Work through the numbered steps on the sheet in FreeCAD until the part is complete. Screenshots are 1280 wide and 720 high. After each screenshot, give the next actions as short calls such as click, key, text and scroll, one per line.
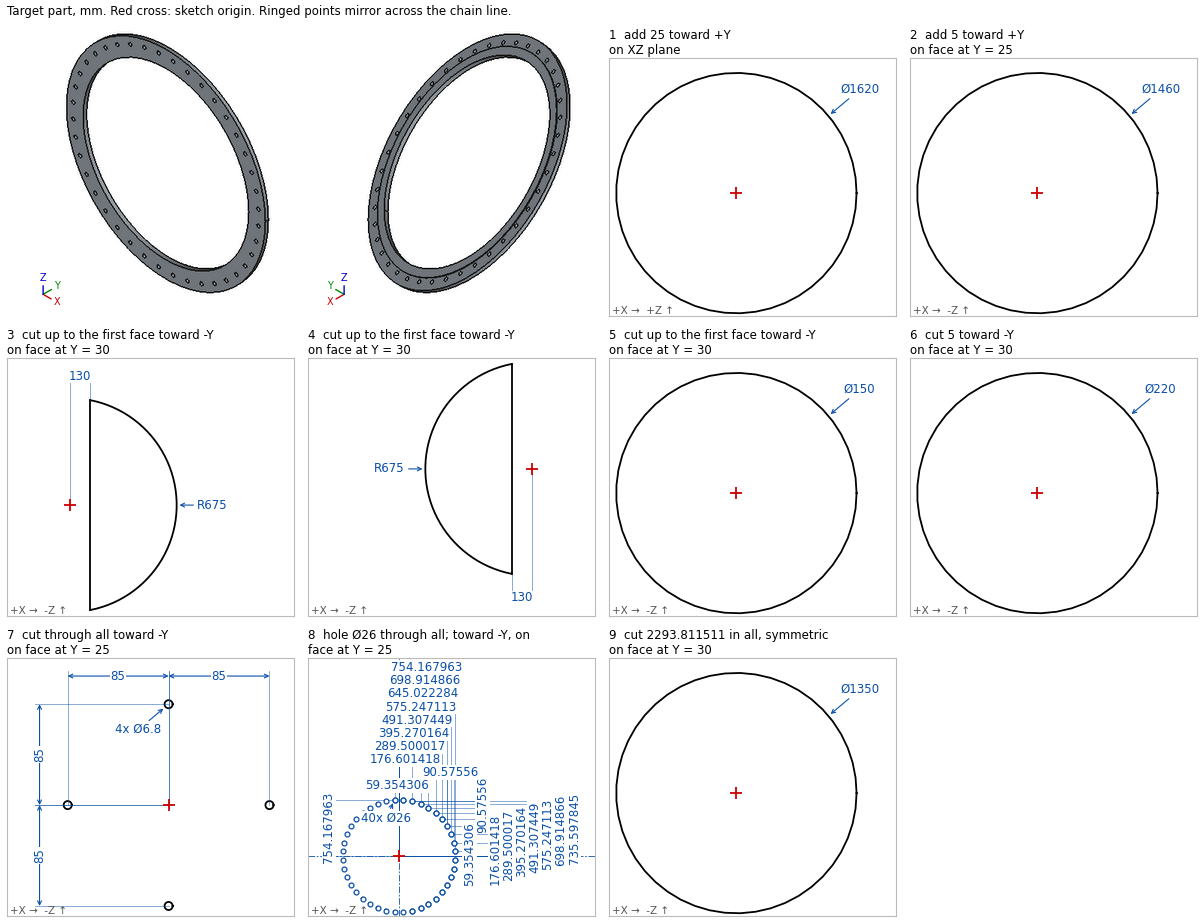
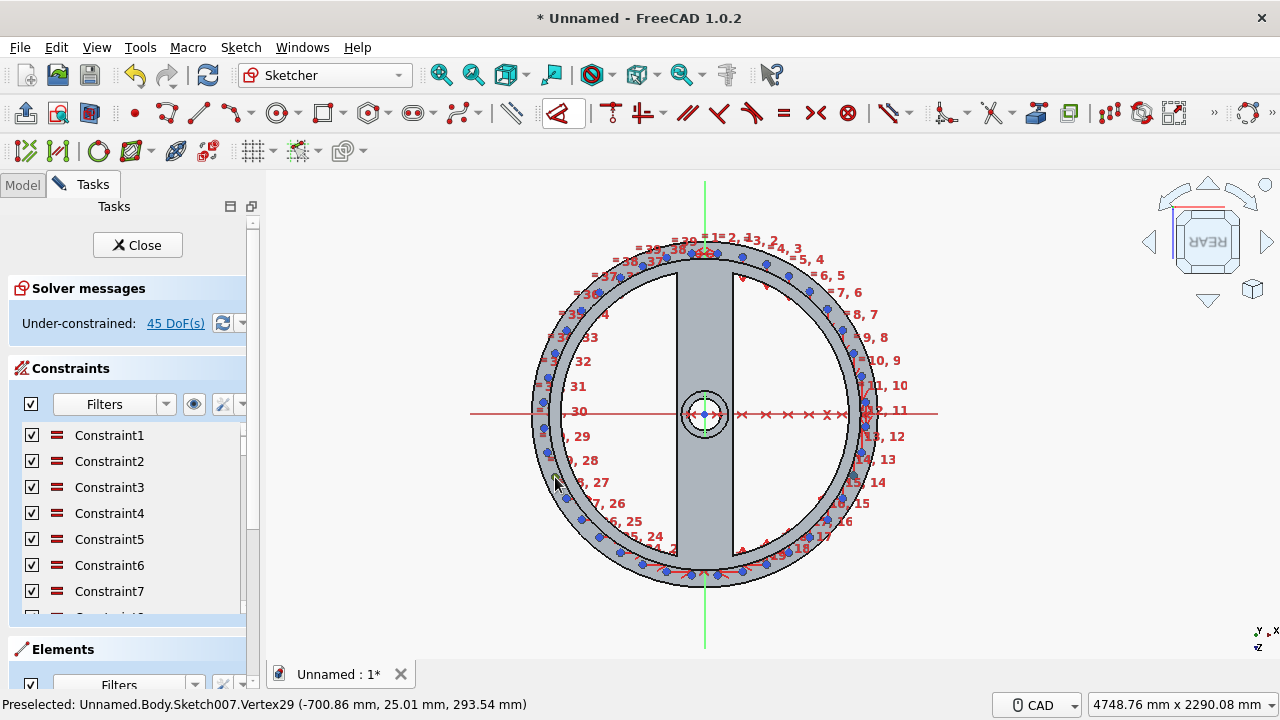
click(705, 507)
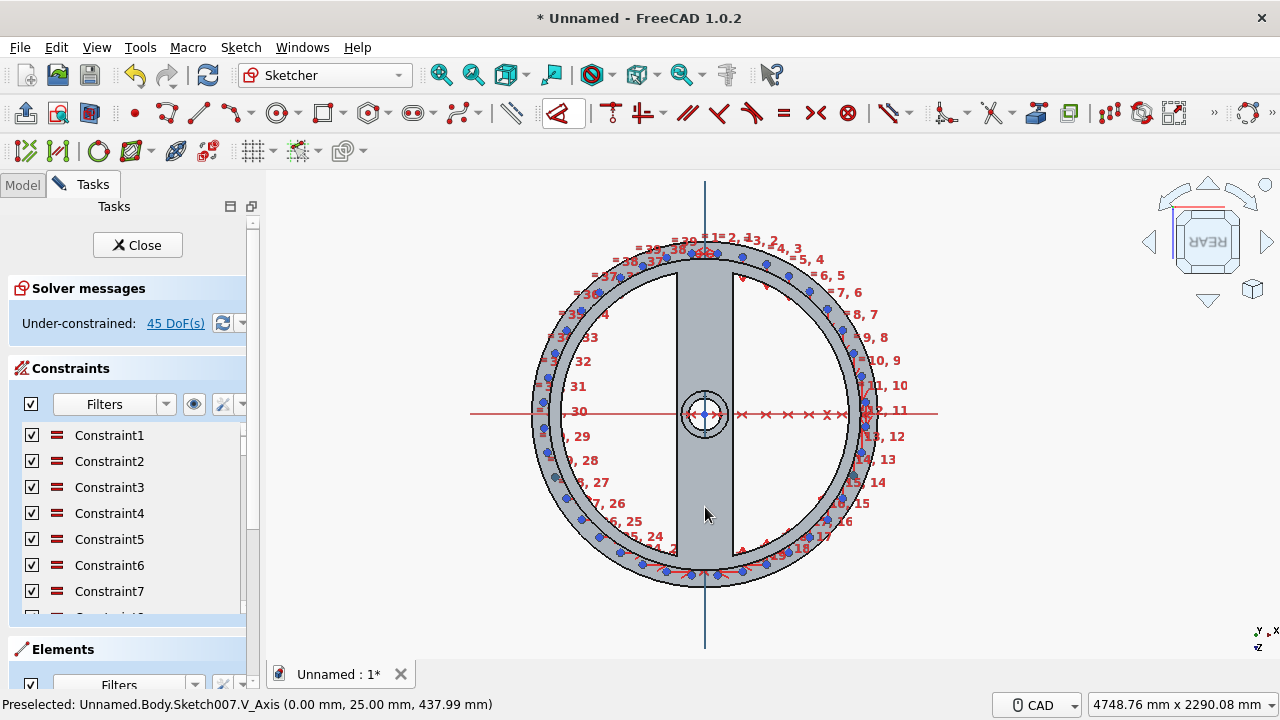
click(816, 114)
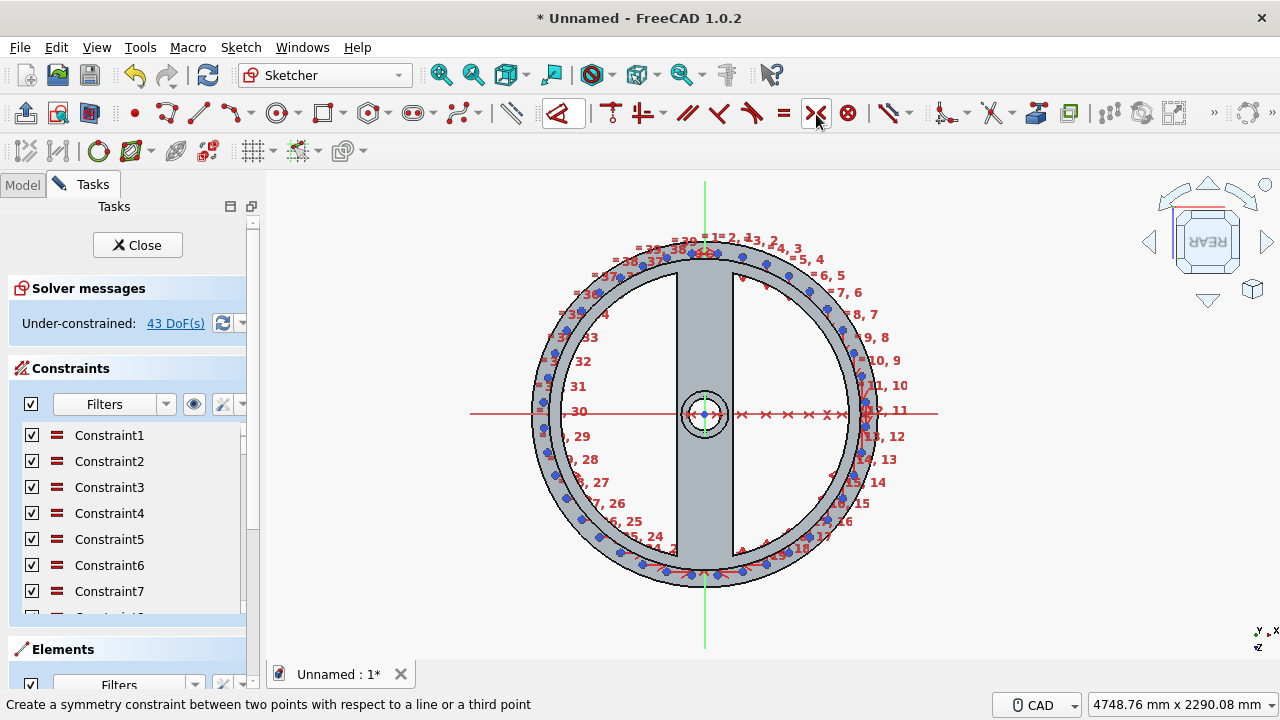
click(862, 453)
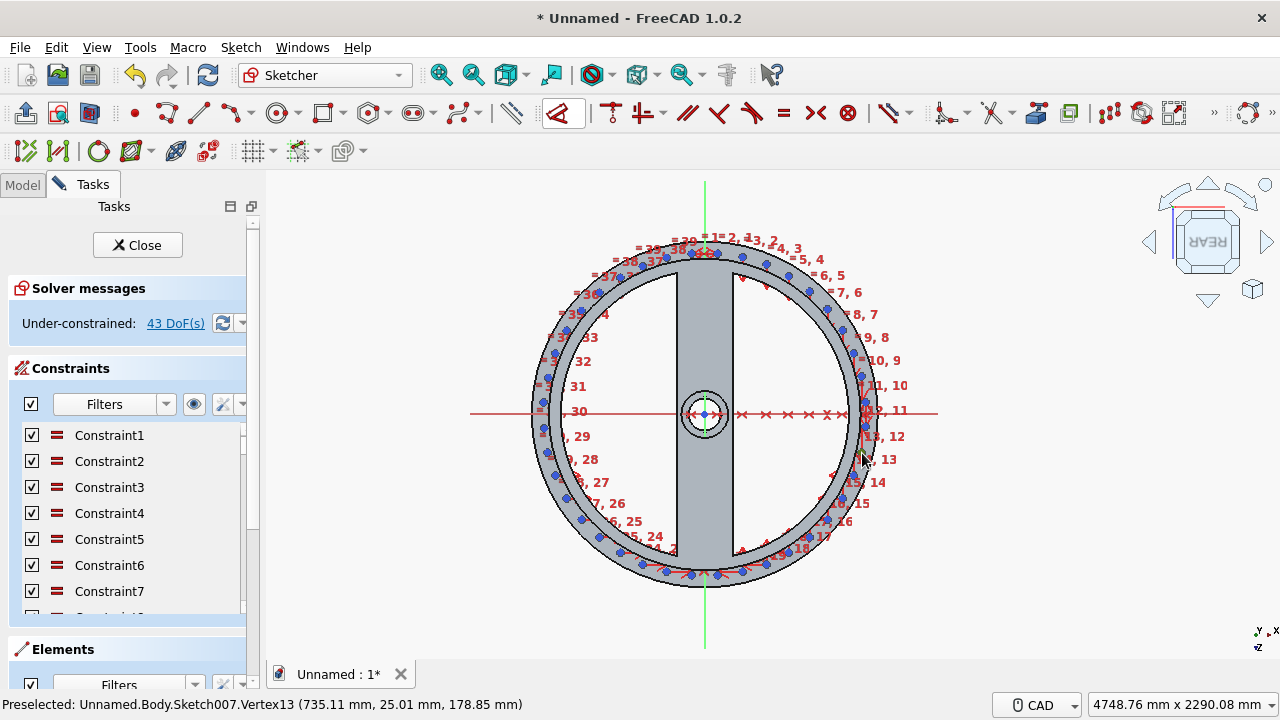
click(548, 453)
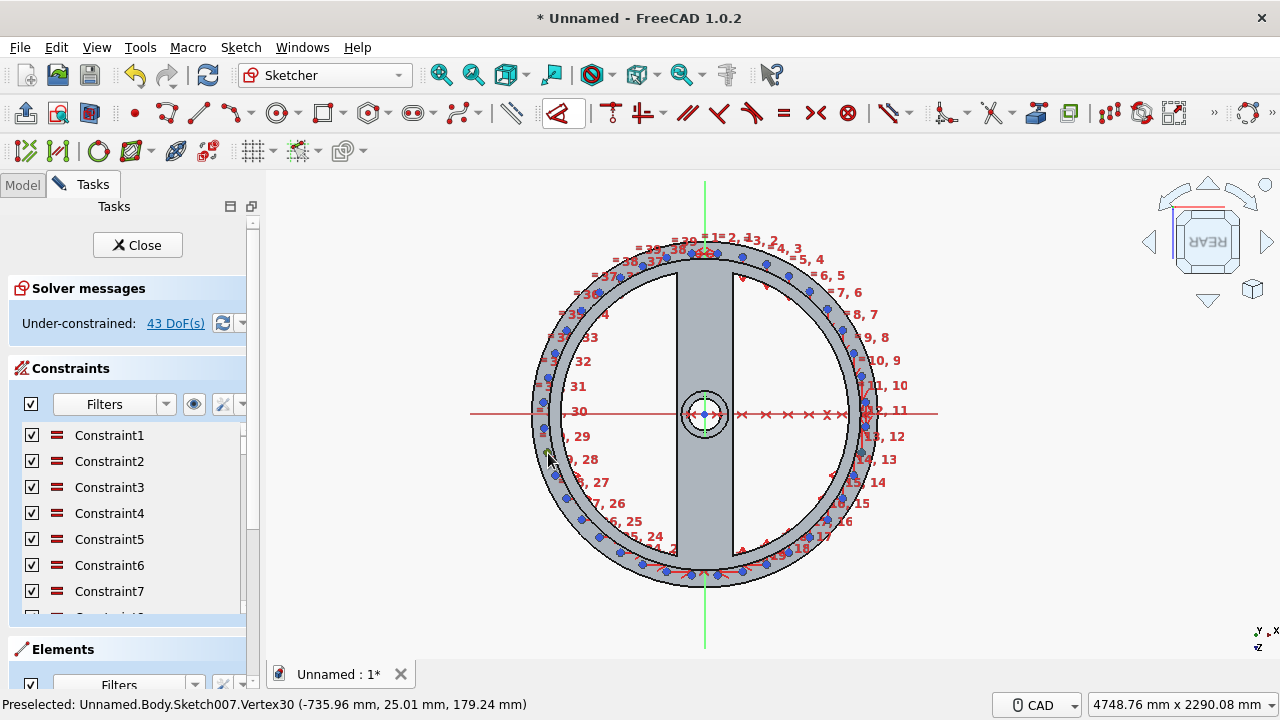
click(705, 507)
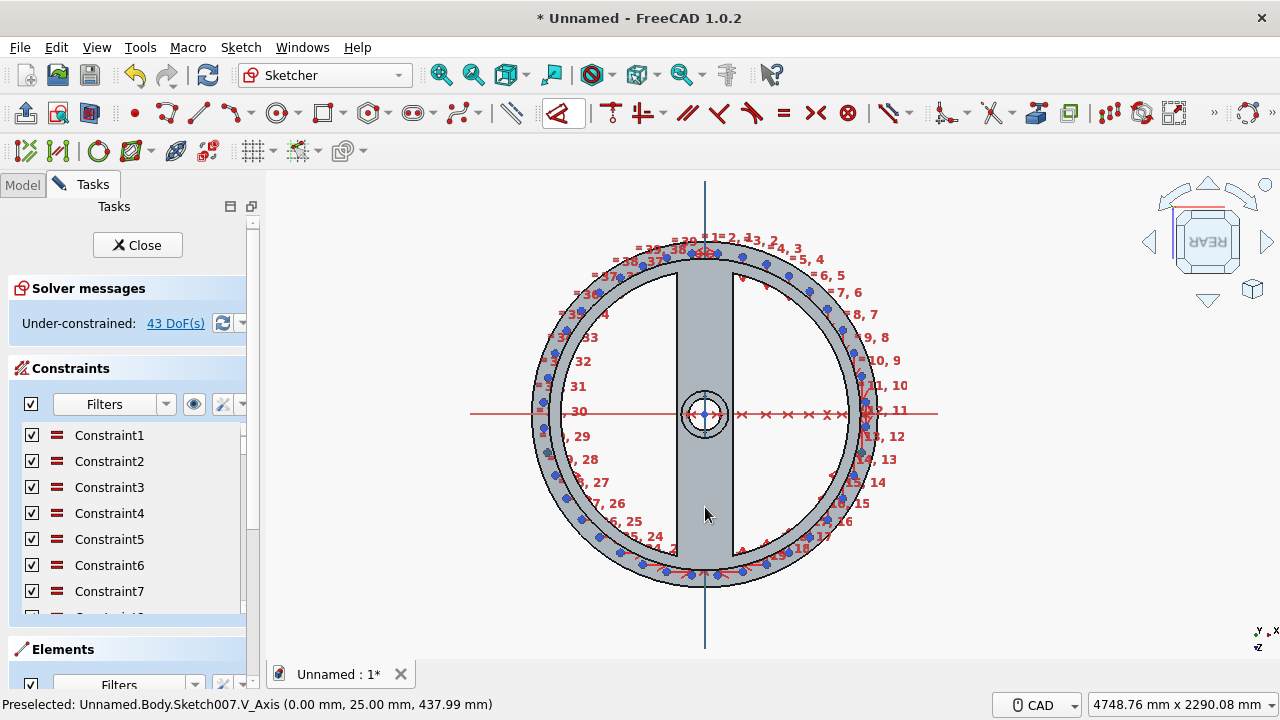
click(816, 114)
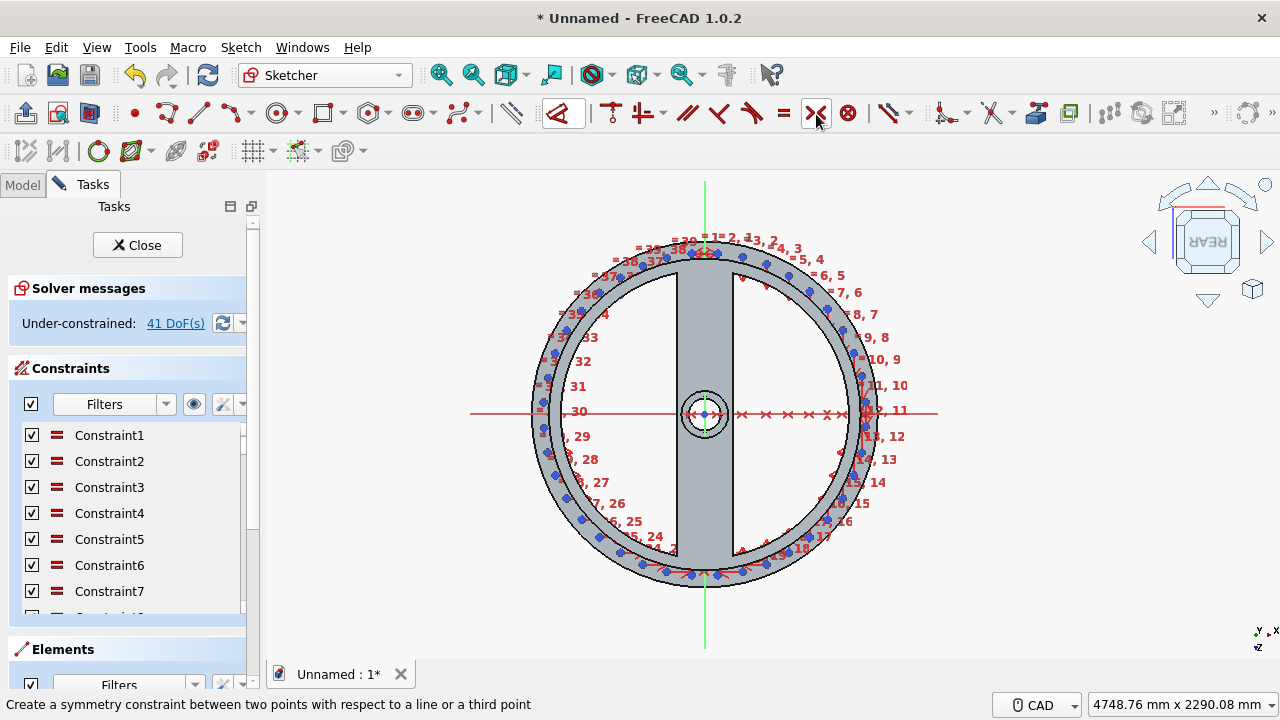
click(866, 427)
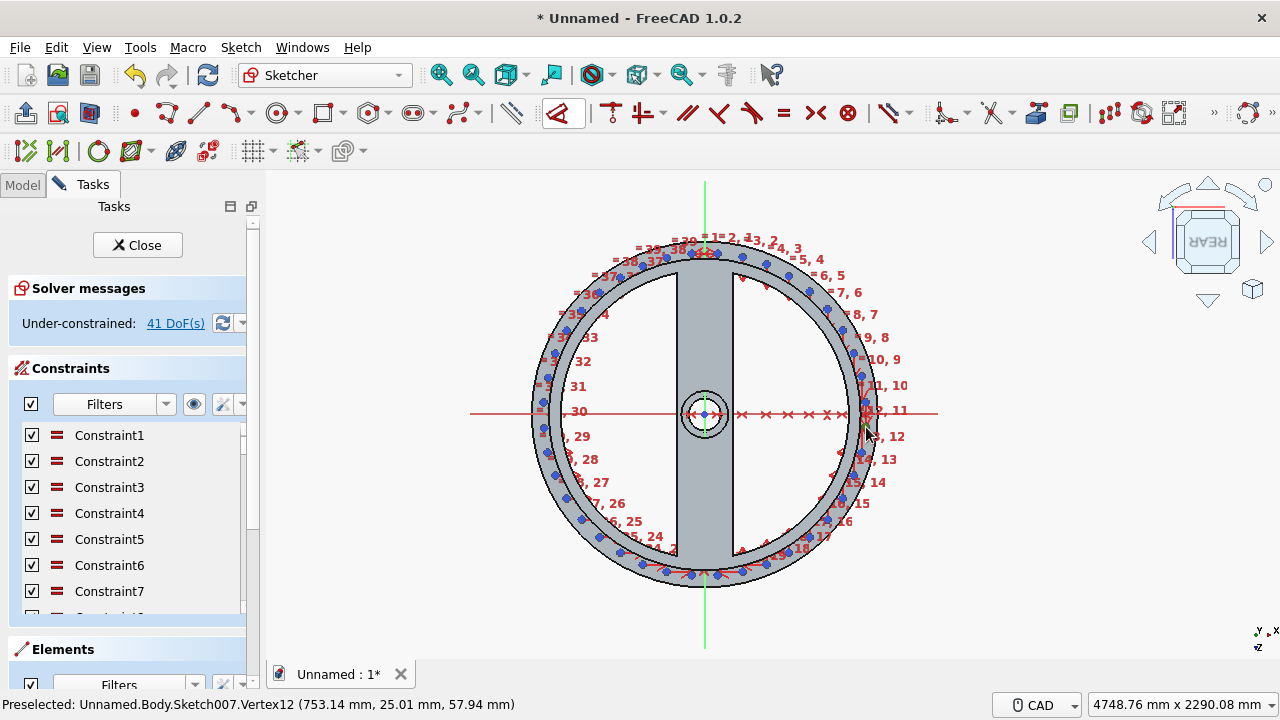
click(544, 428)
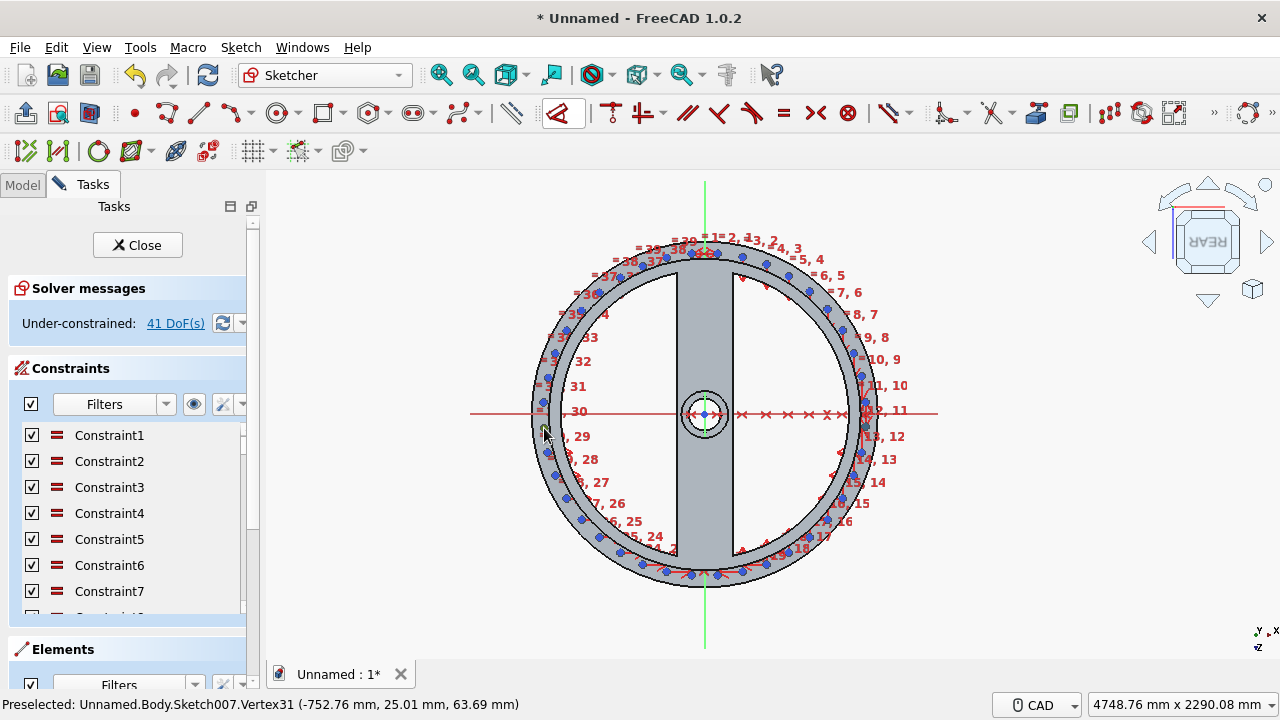
click(705, 507)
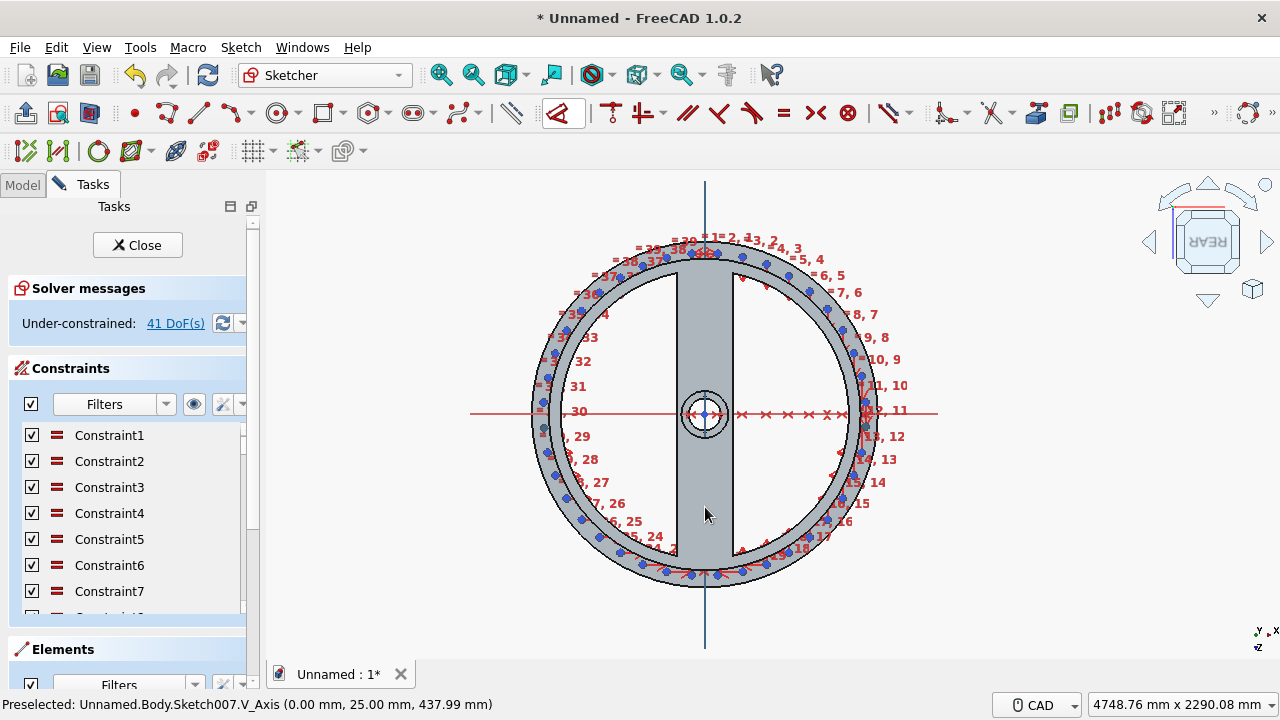
click(816, 114)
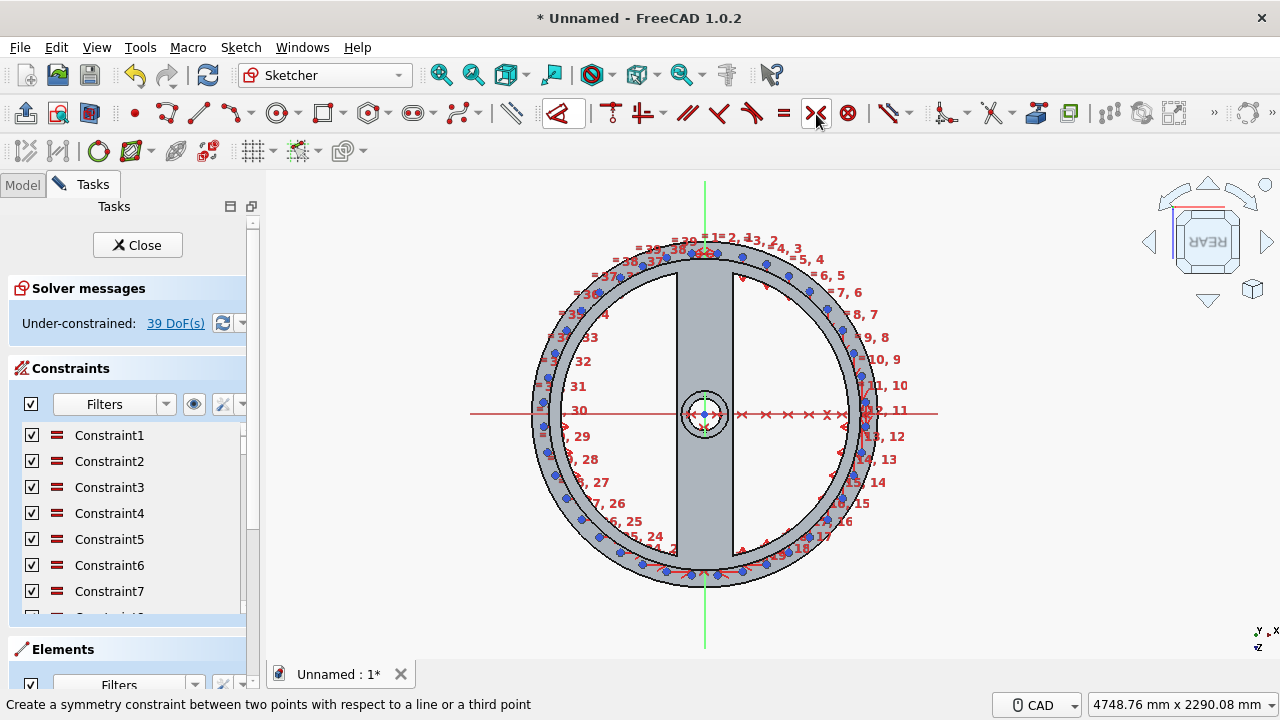
click(866, 402)